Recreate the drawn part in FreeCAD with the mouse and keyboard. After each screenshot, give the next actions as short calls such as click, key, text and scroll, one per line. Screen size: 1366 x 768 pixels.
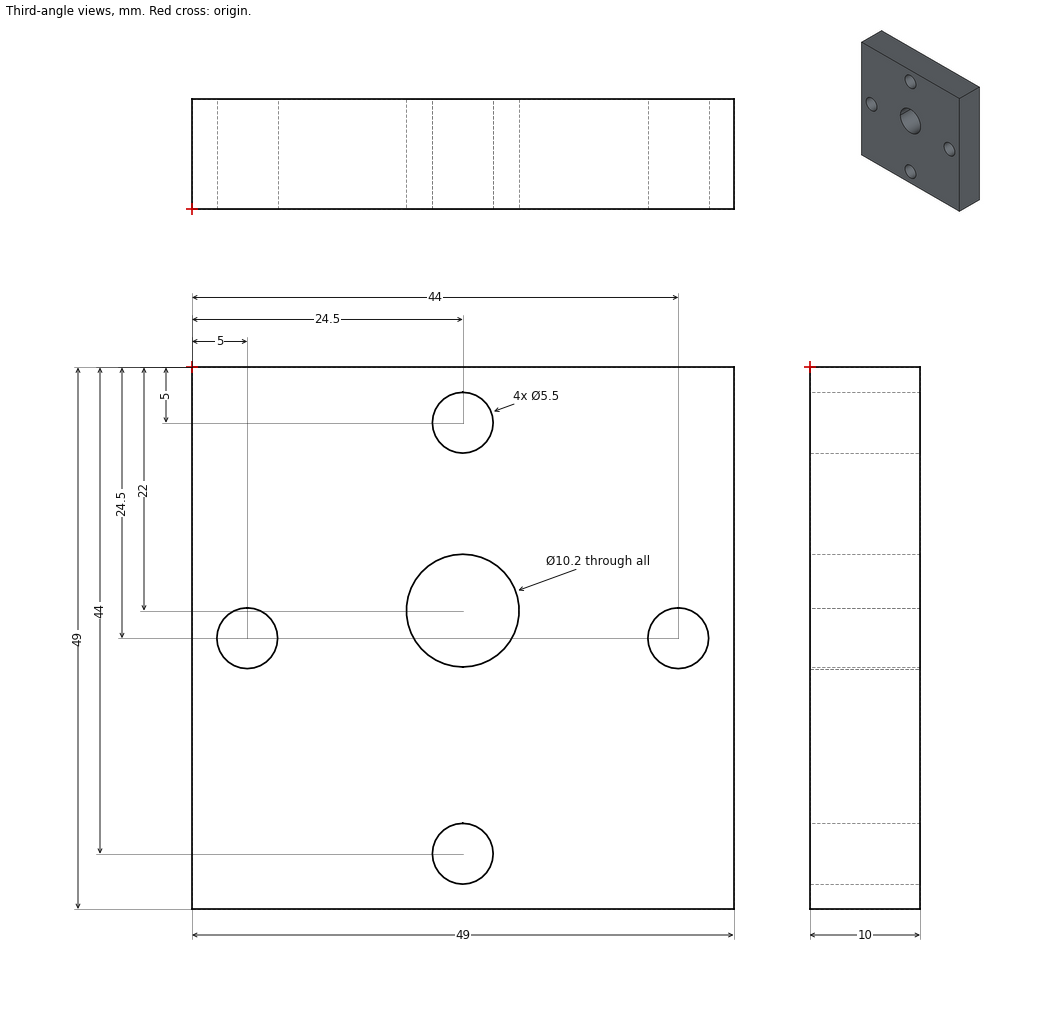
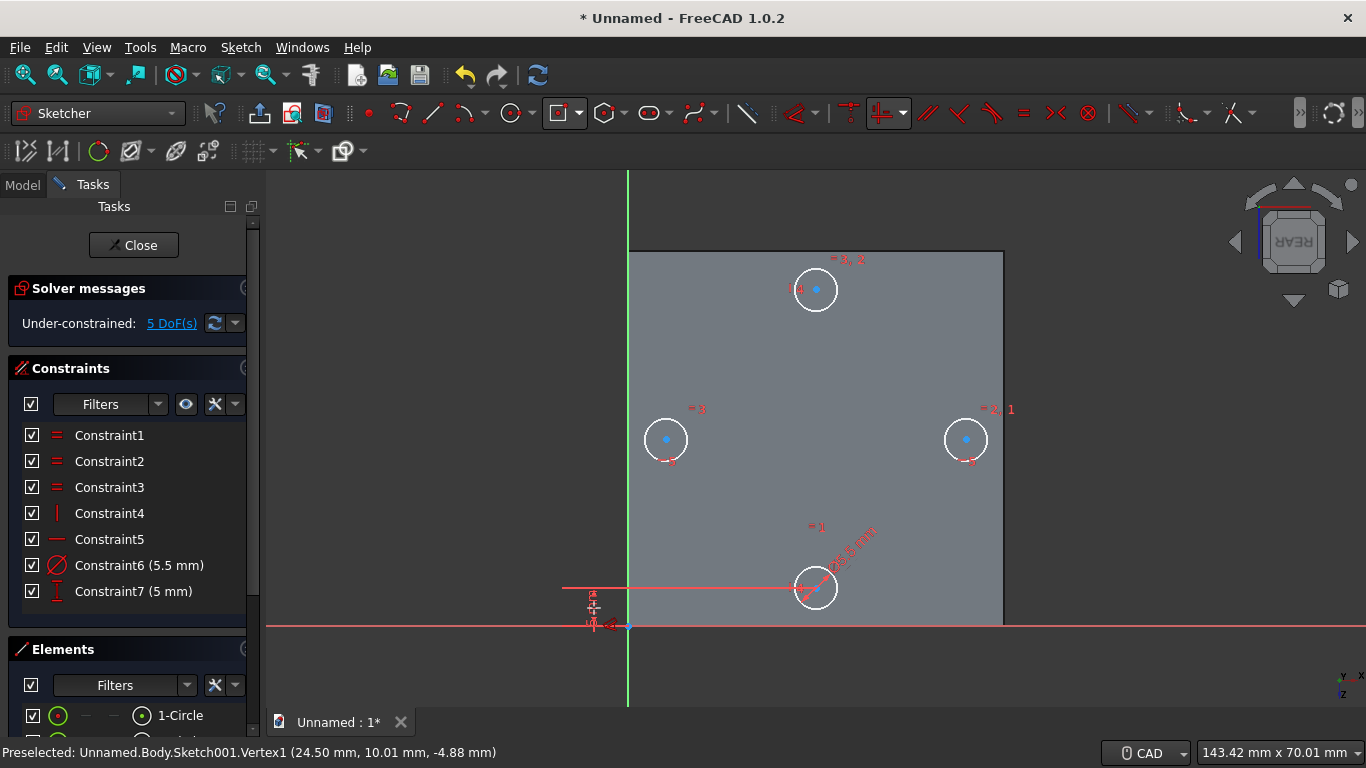
click(666, 440)
click(647, 660)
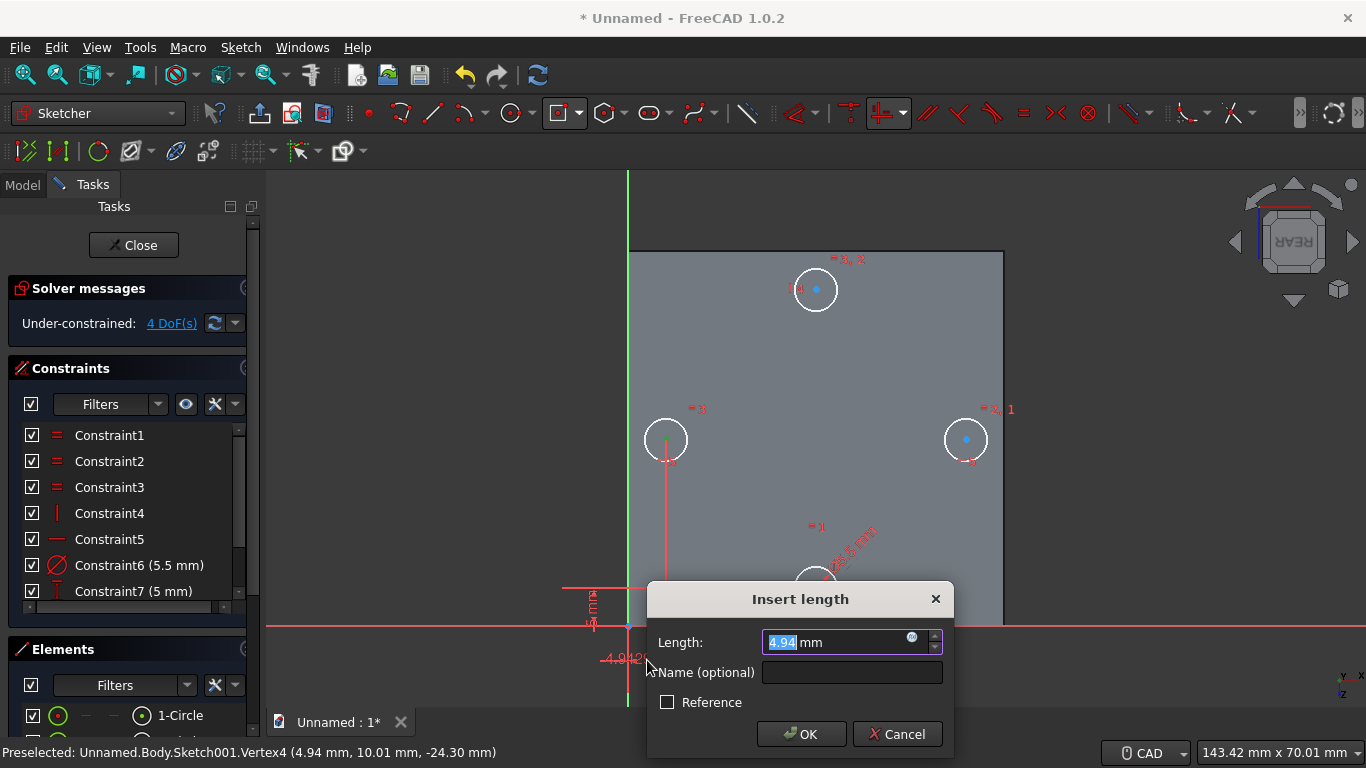
text(5)
key(Return)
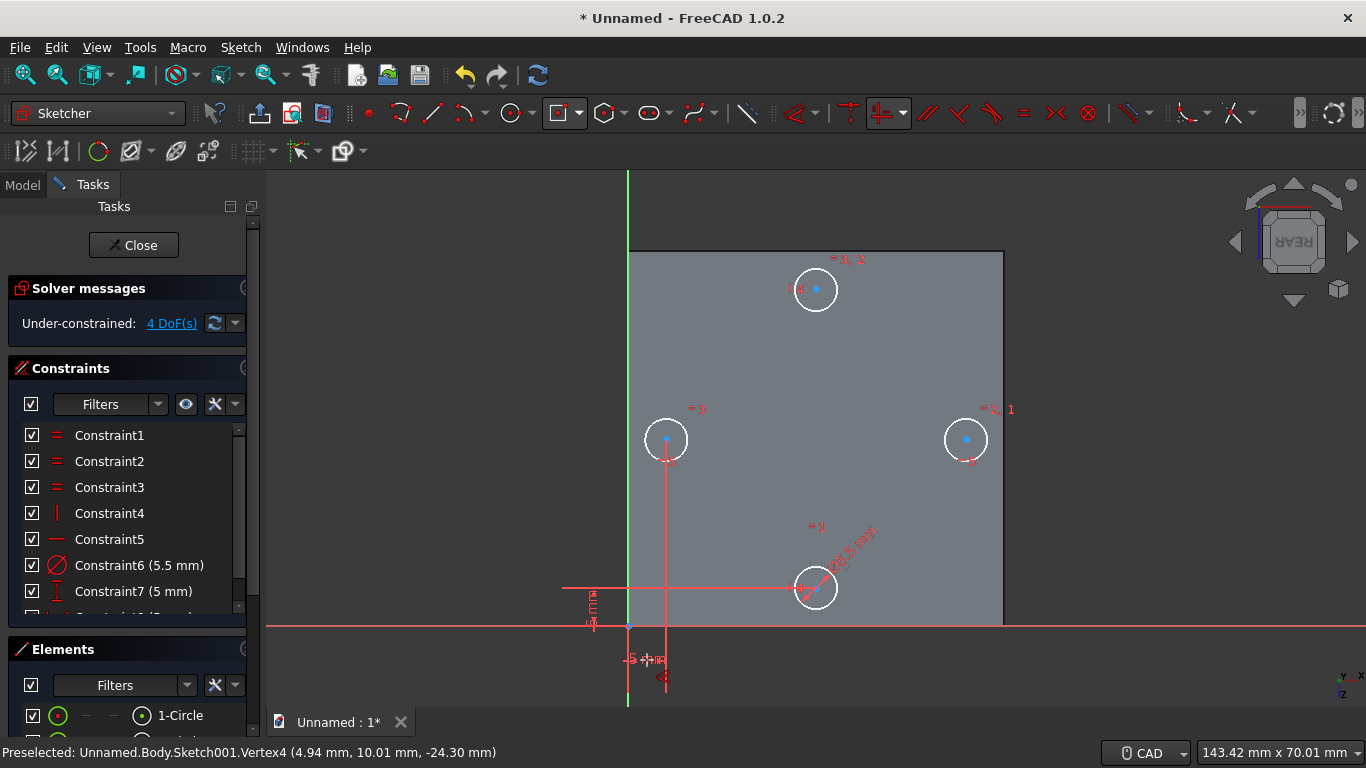
click(966, 440)
click(797, 660)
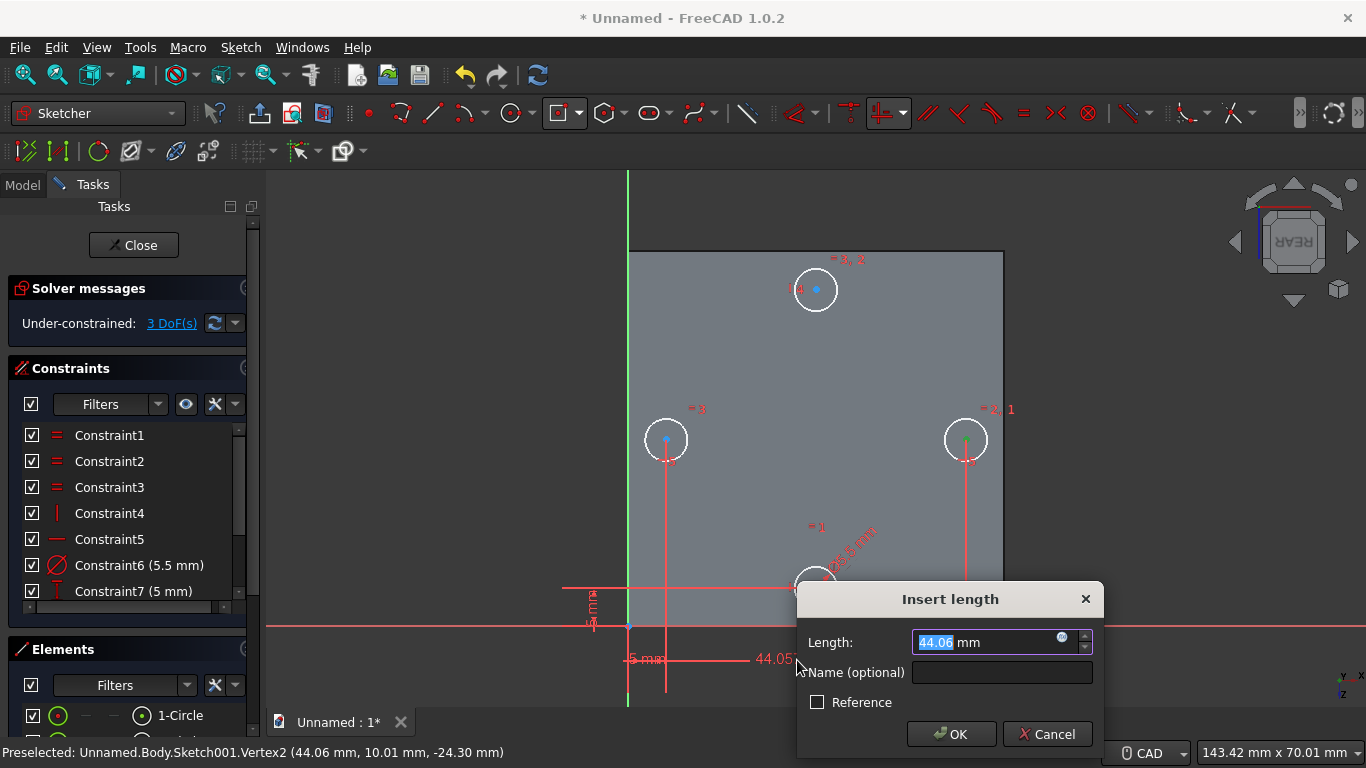
text(44)
key(Return)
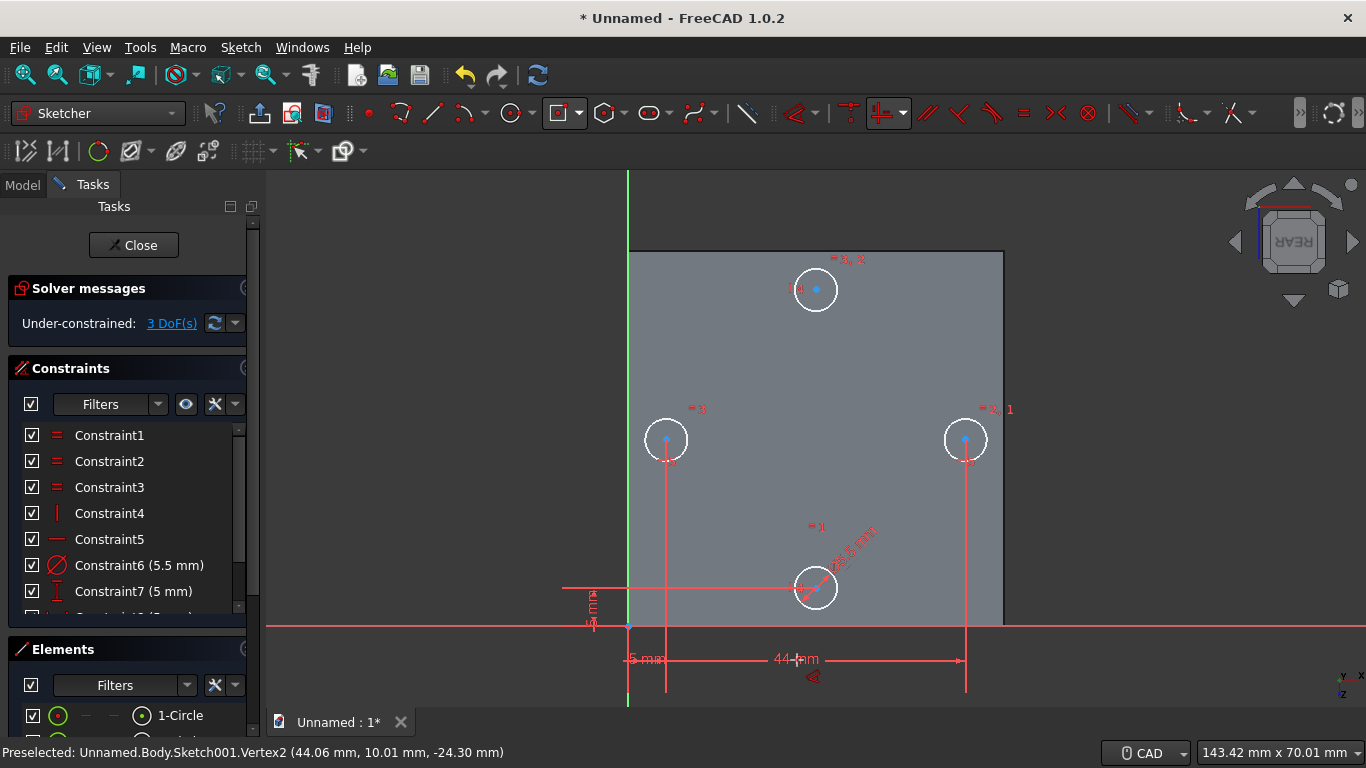
click(816, 290)
click(594, 458)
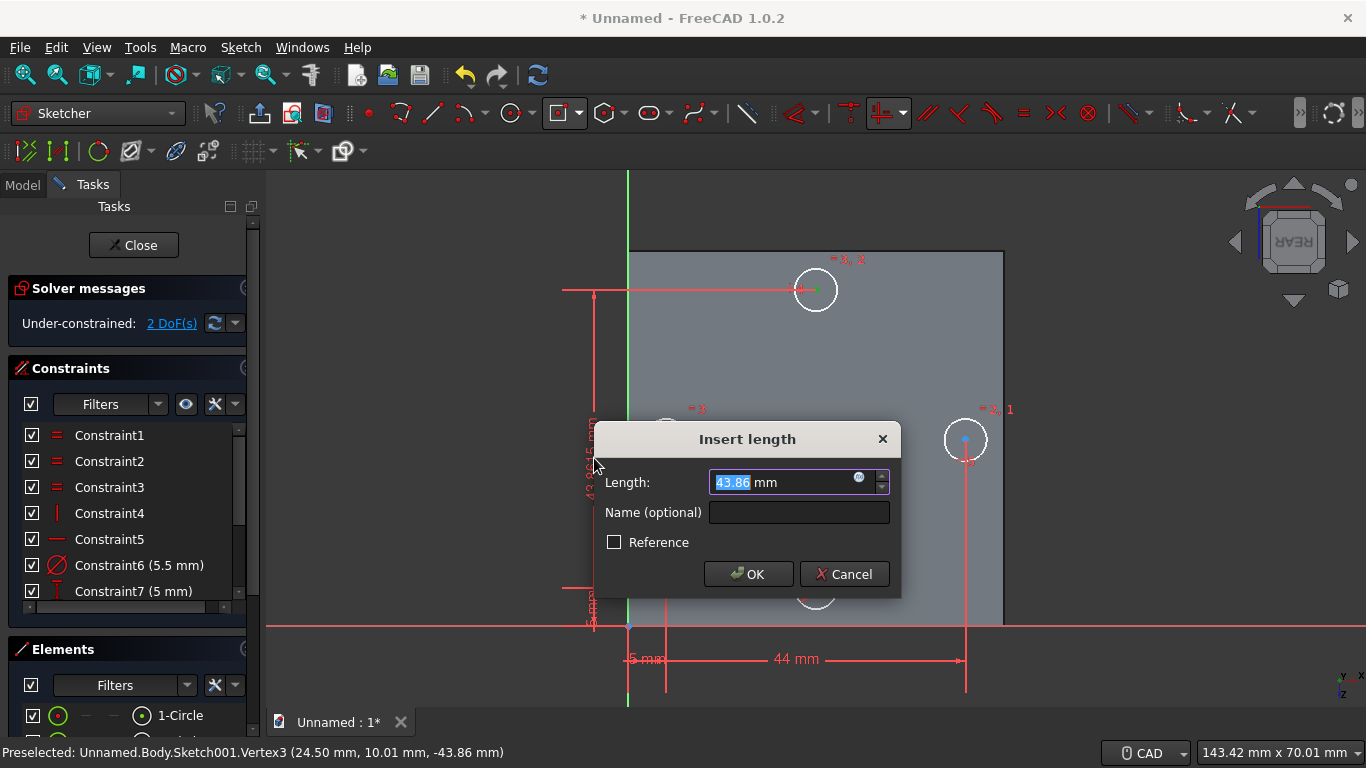
text(44)
key(Return)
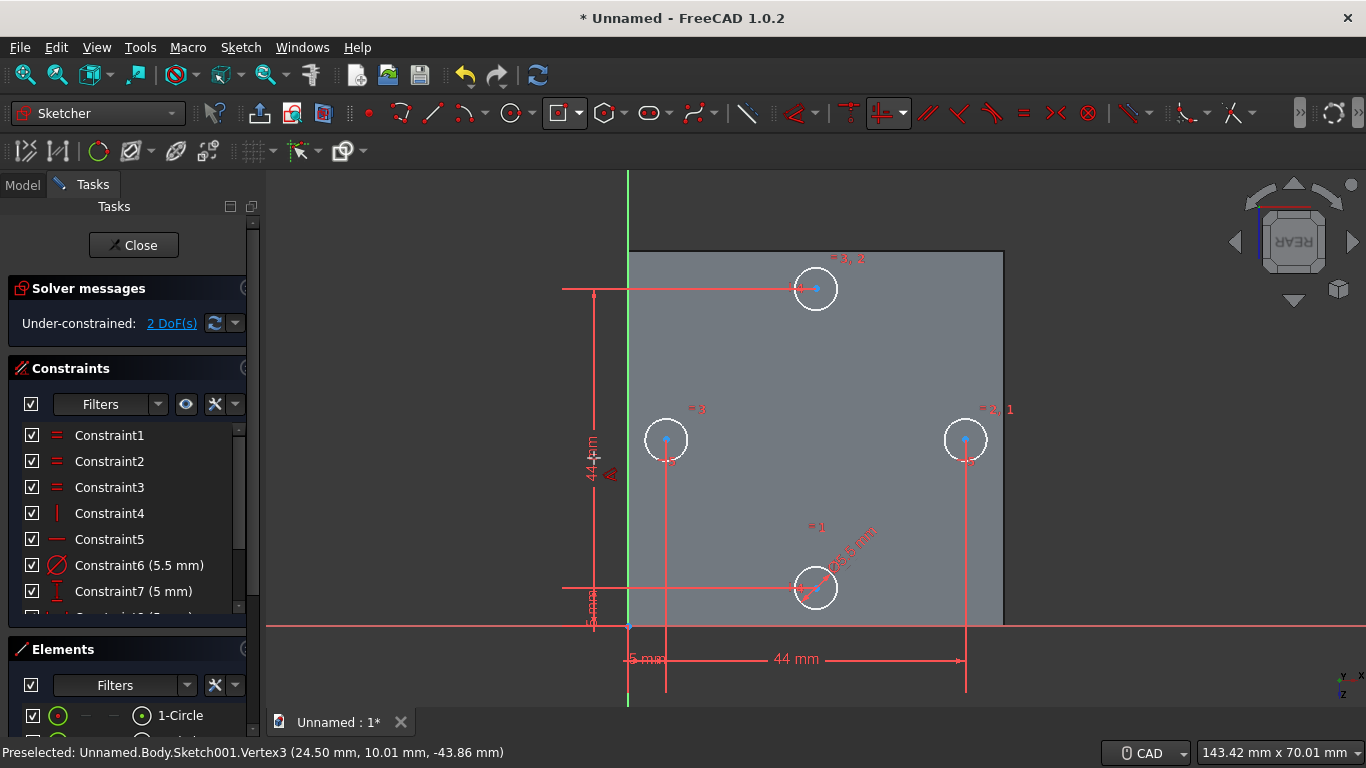
click(816, 588)
click(722, 660)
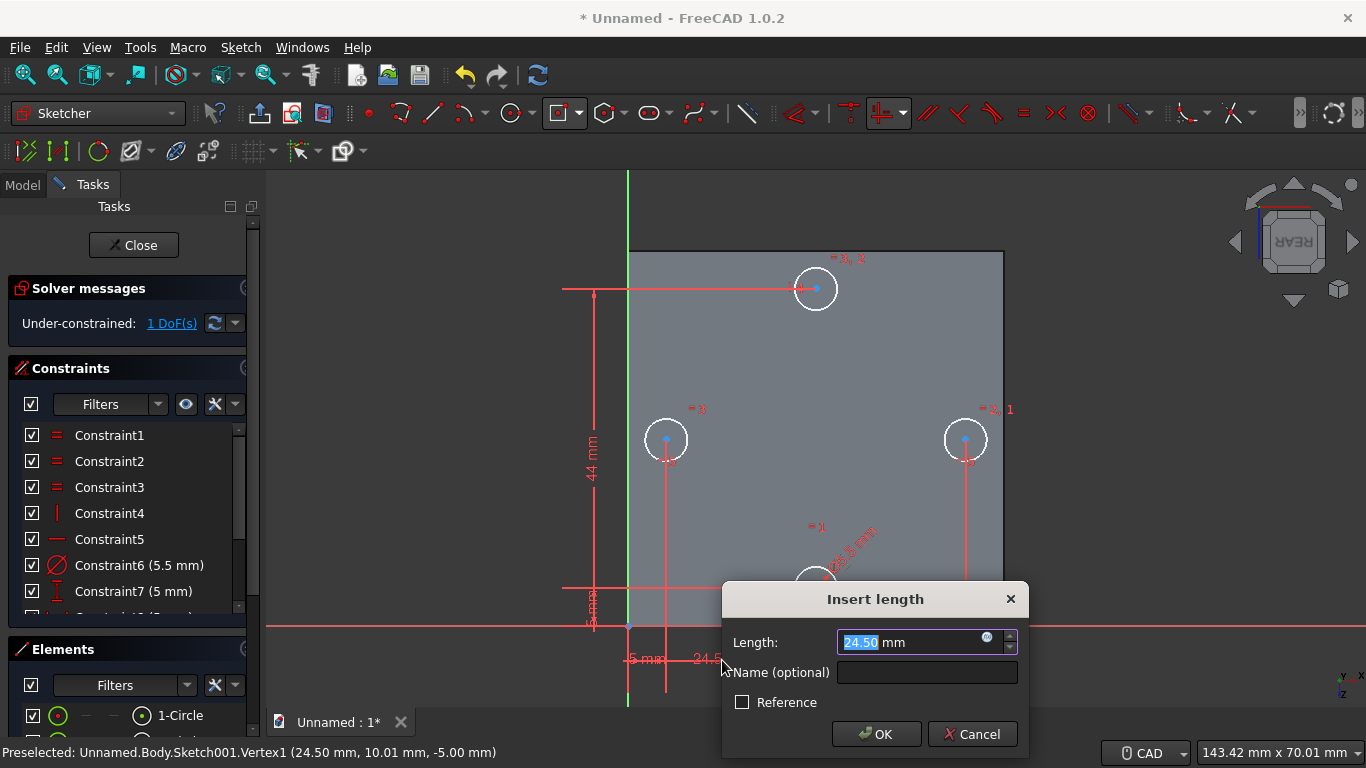
text(24.5)
key(Return)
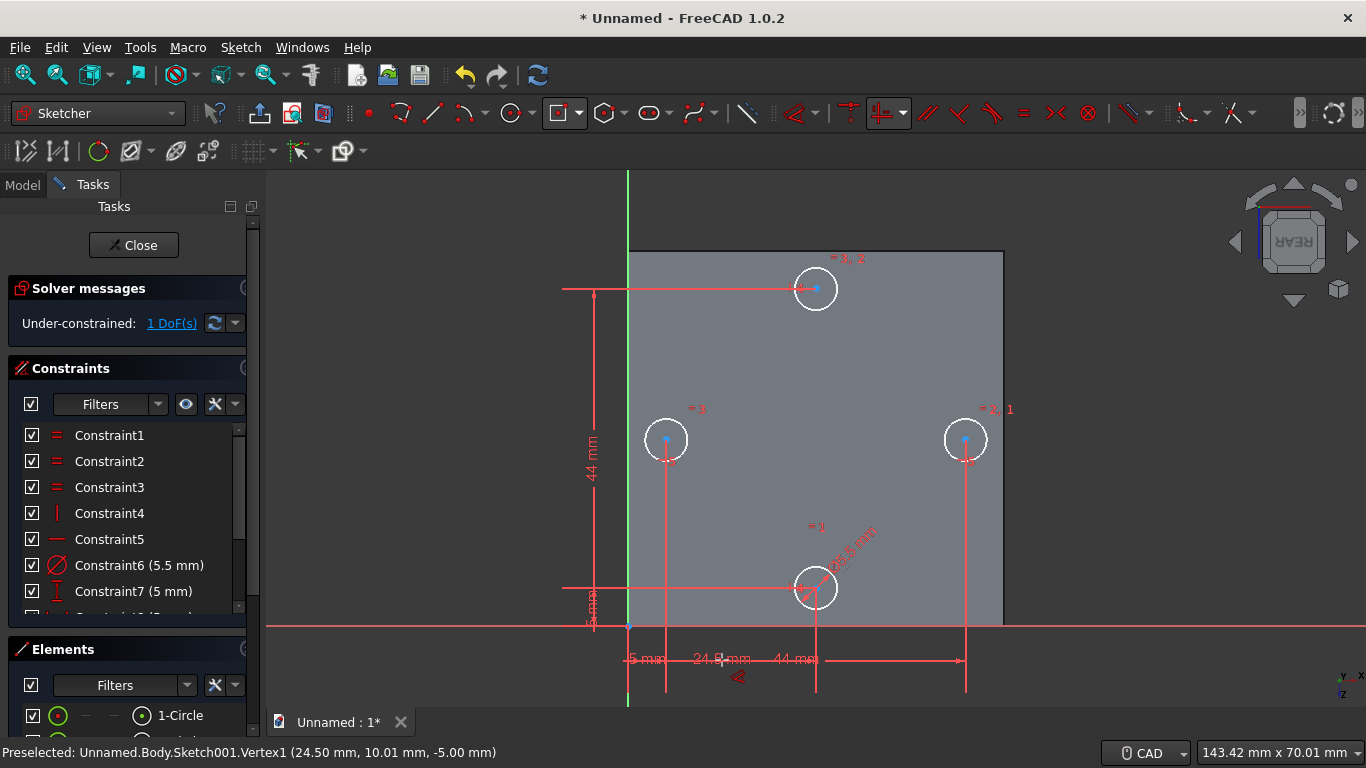
click(966, 440)
click(594, 533)